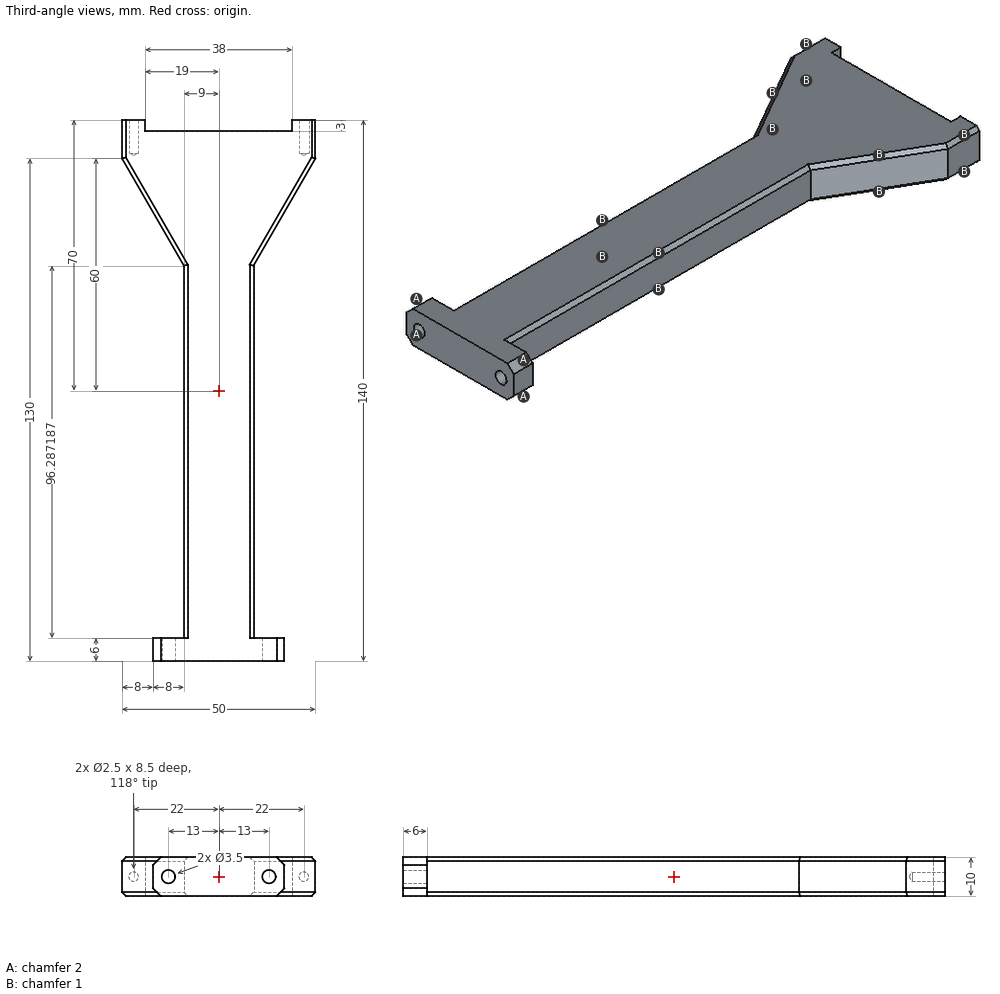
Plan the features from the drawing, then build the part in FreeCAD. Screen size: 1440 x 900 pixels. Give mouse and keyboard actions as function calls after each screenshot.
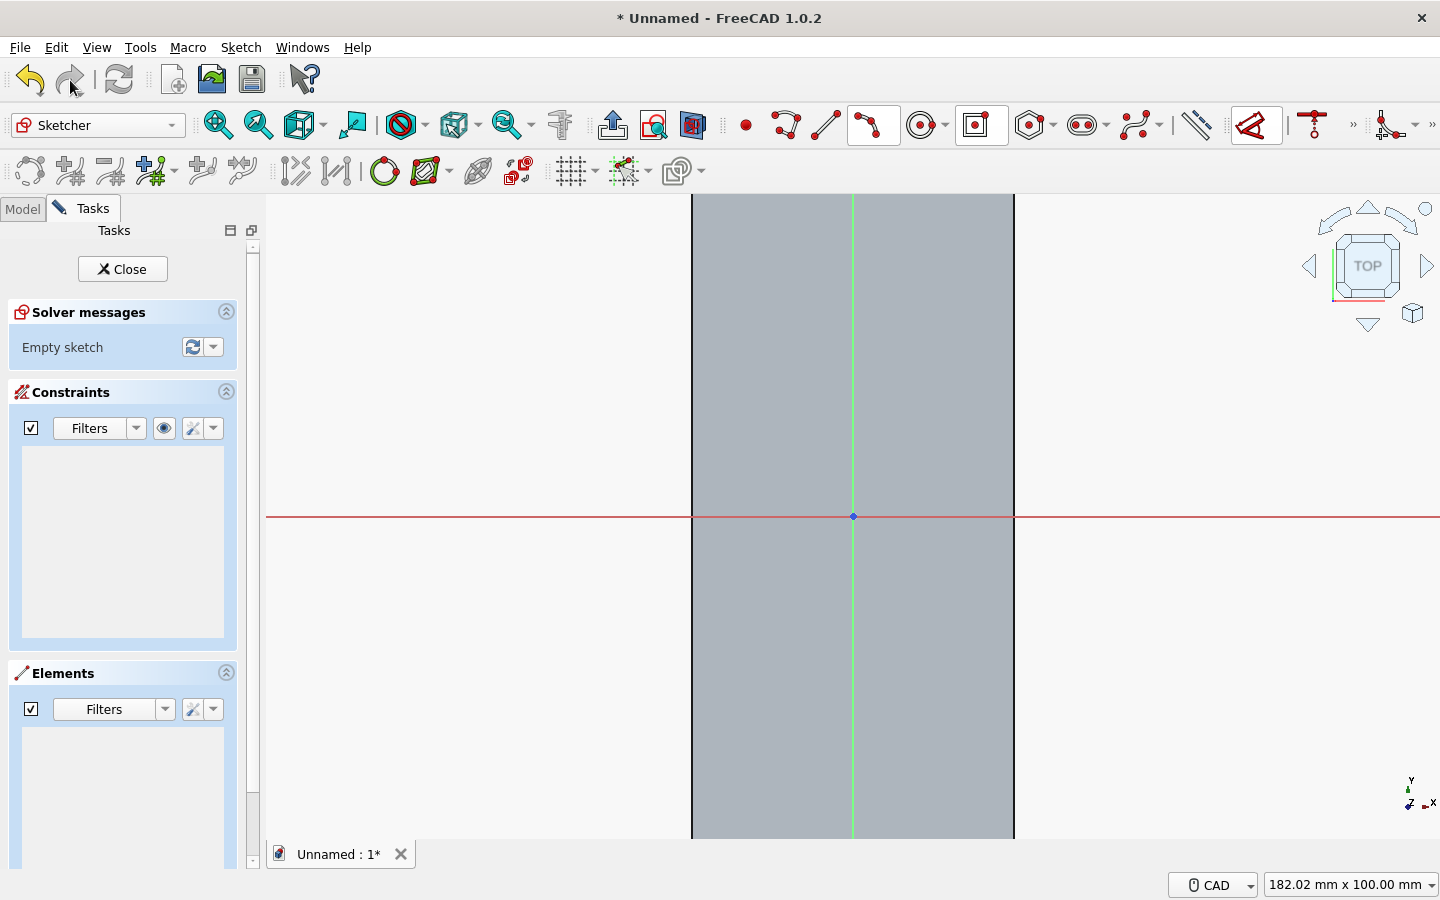
scroll(794, 490, down, 4)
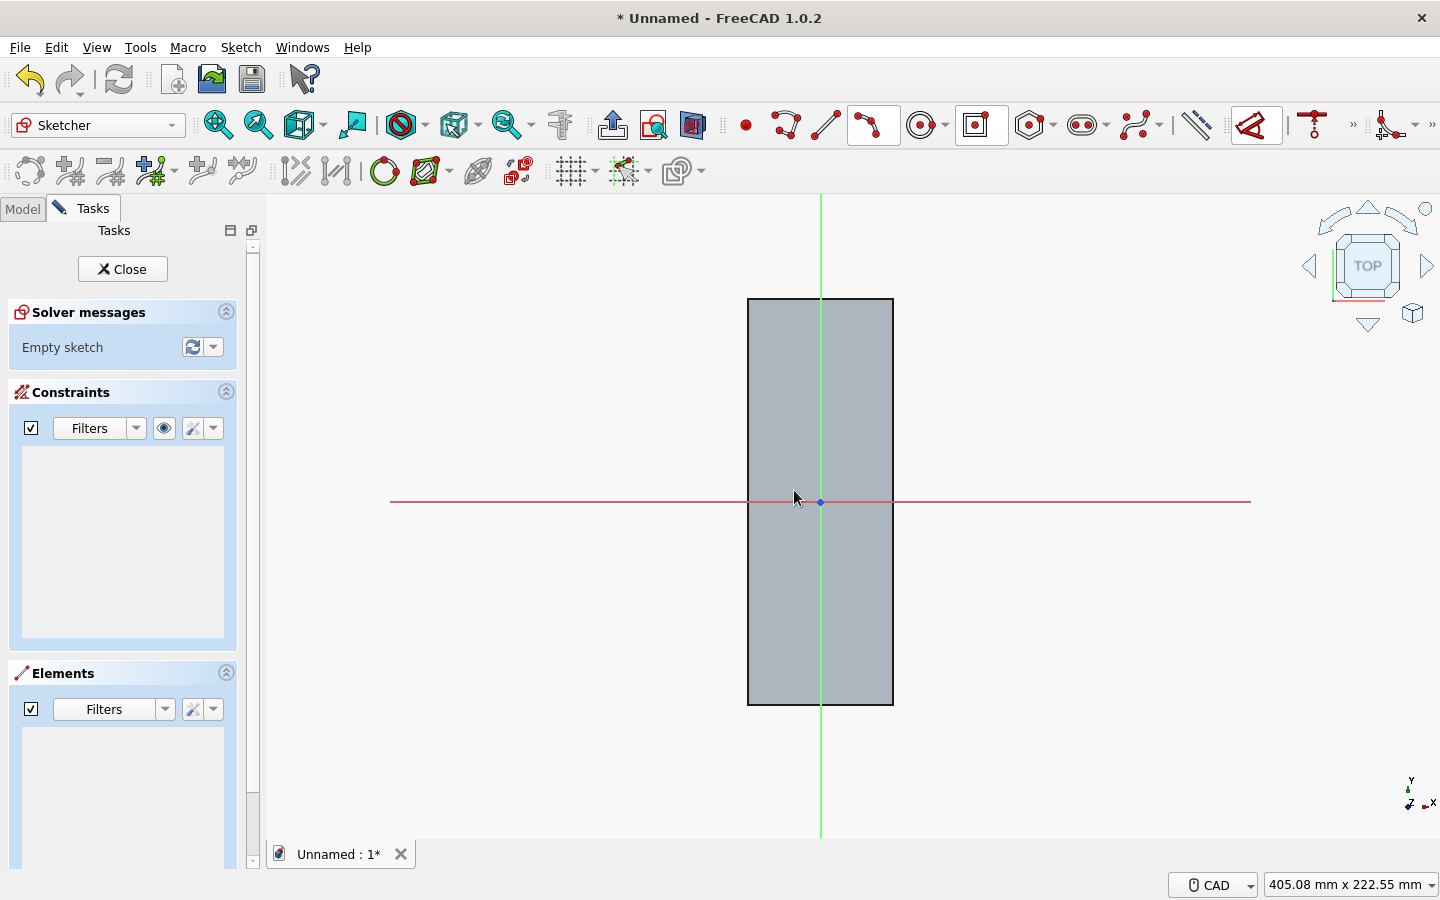
click(786, 126)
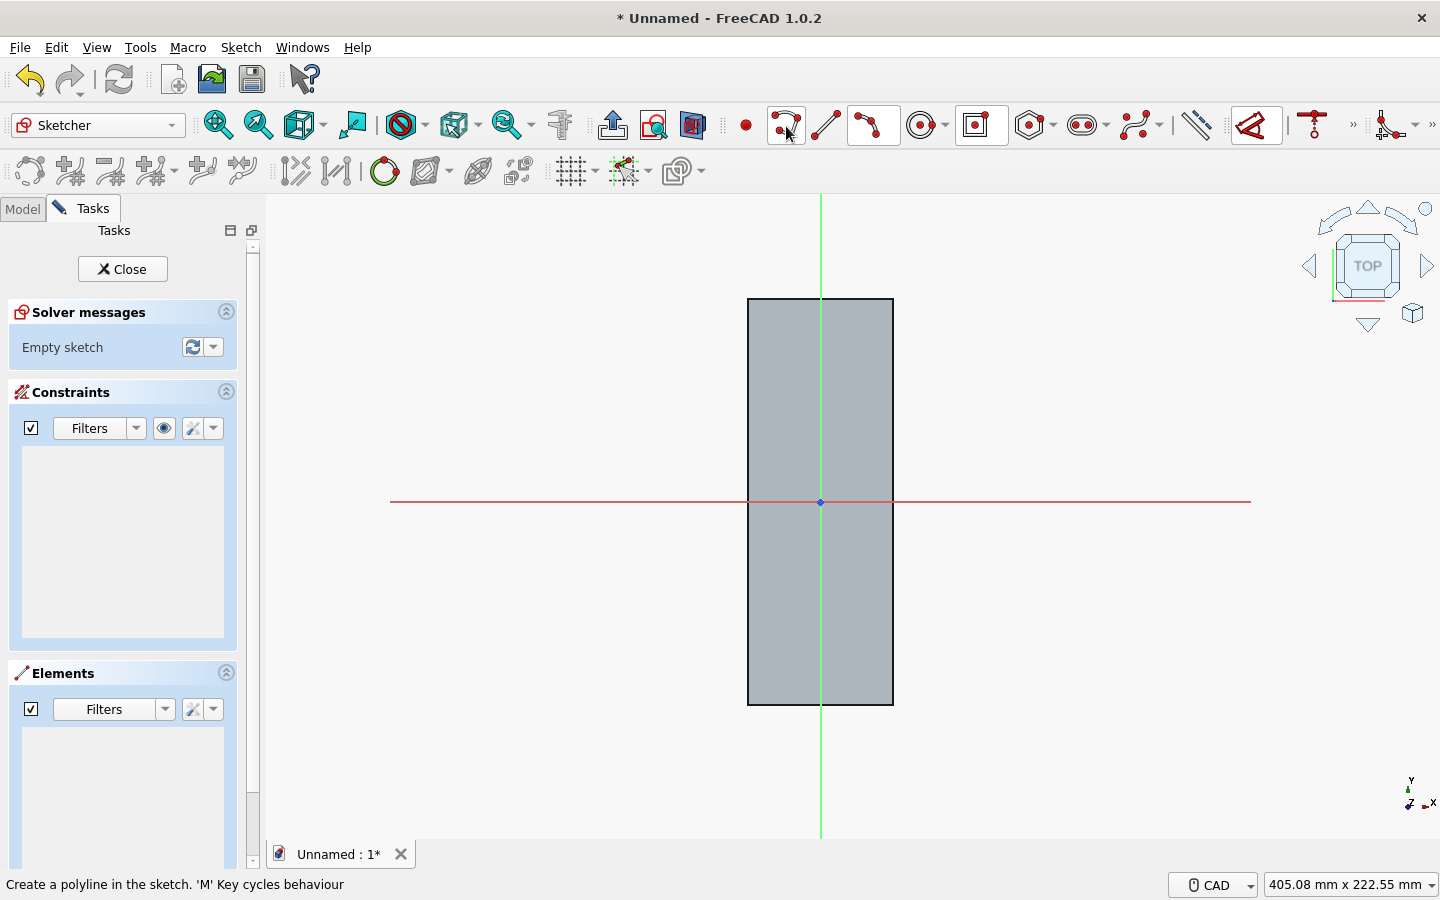
click(795, 409)
click(748, 328)
click(748, 705)
click(771, 705)
click(771, 688)
click(795, 688)
click(795, 410)
key(Escape)
key(Escape)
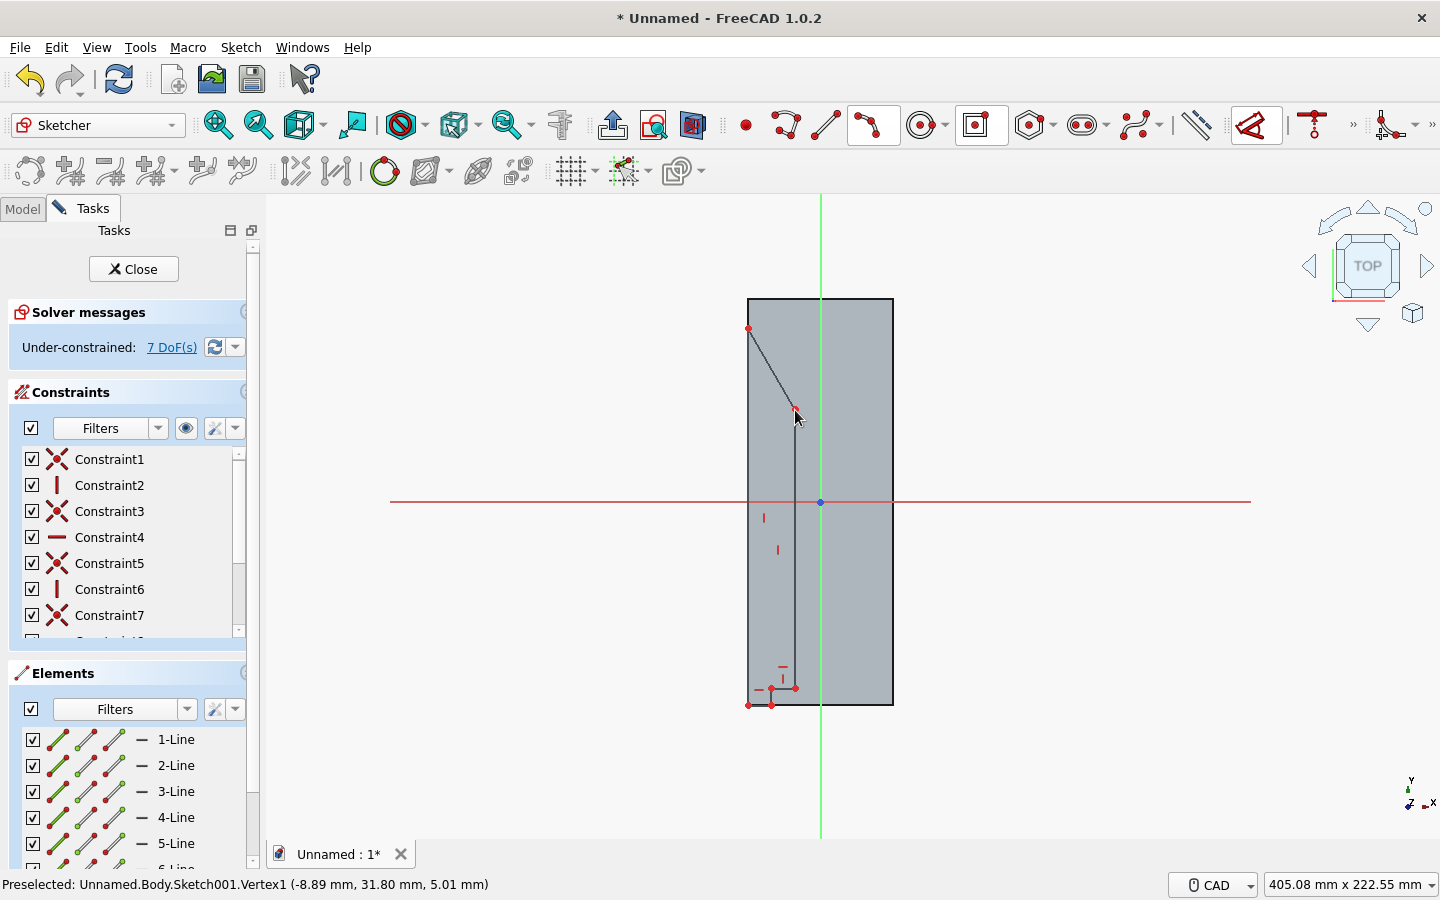
scroll(757, 706, up, 3)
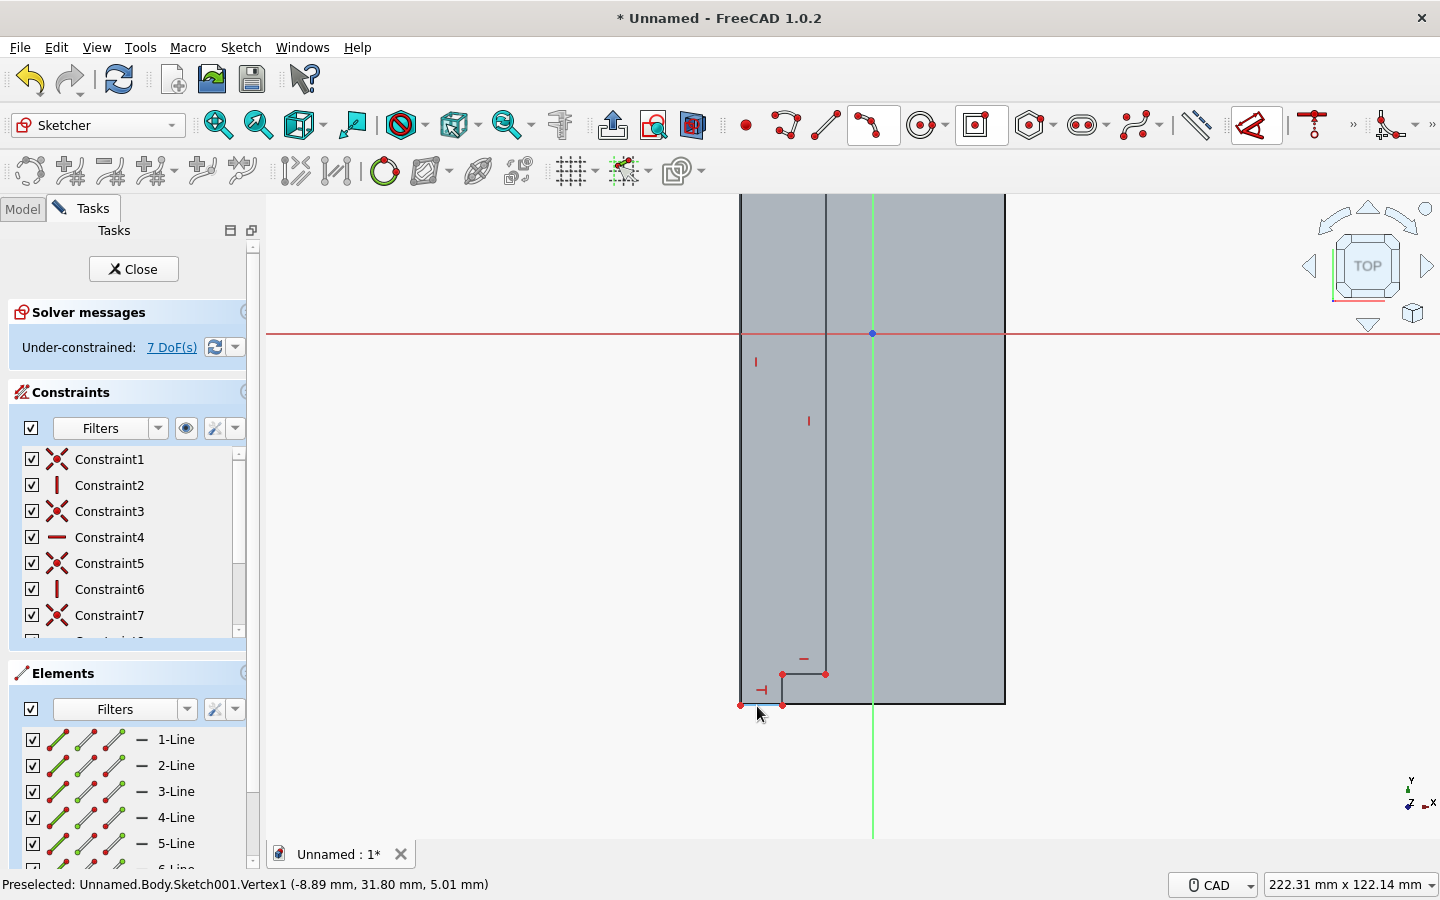
click(757, 705)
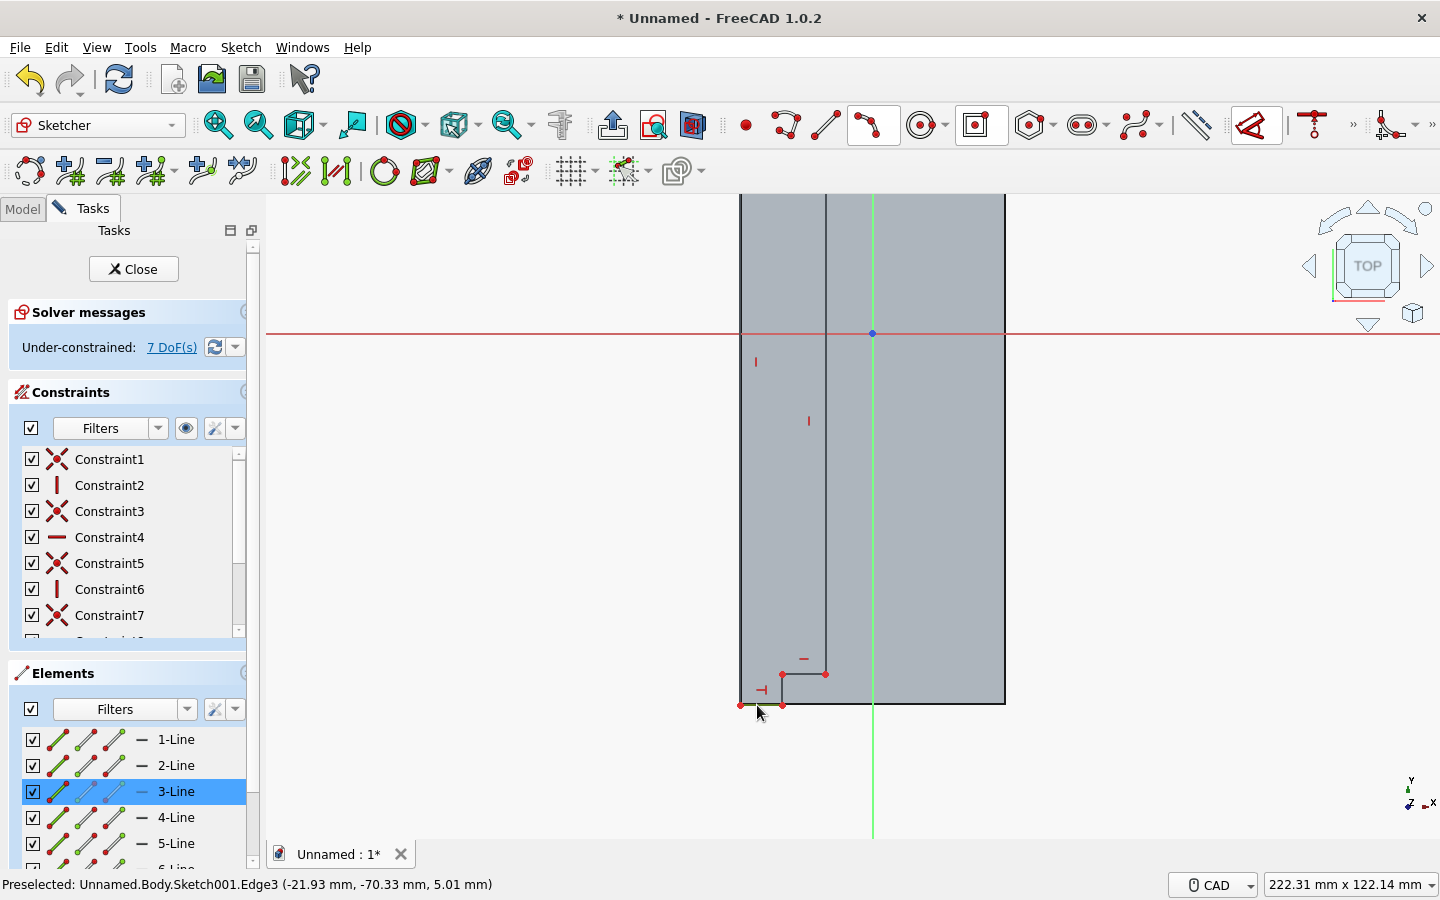
click(1276, 126)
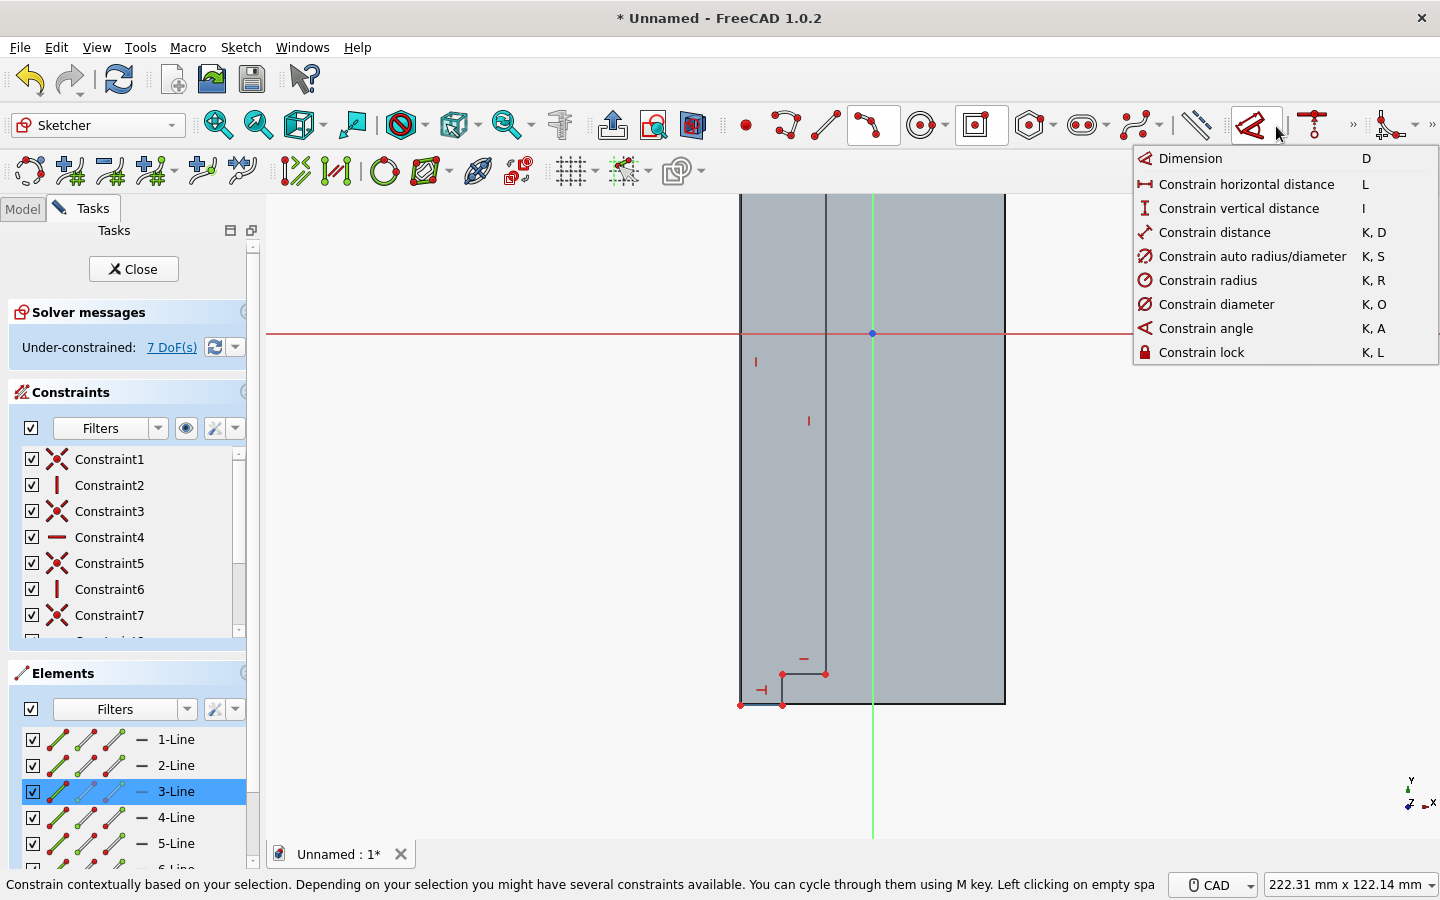
click(1286, 184)